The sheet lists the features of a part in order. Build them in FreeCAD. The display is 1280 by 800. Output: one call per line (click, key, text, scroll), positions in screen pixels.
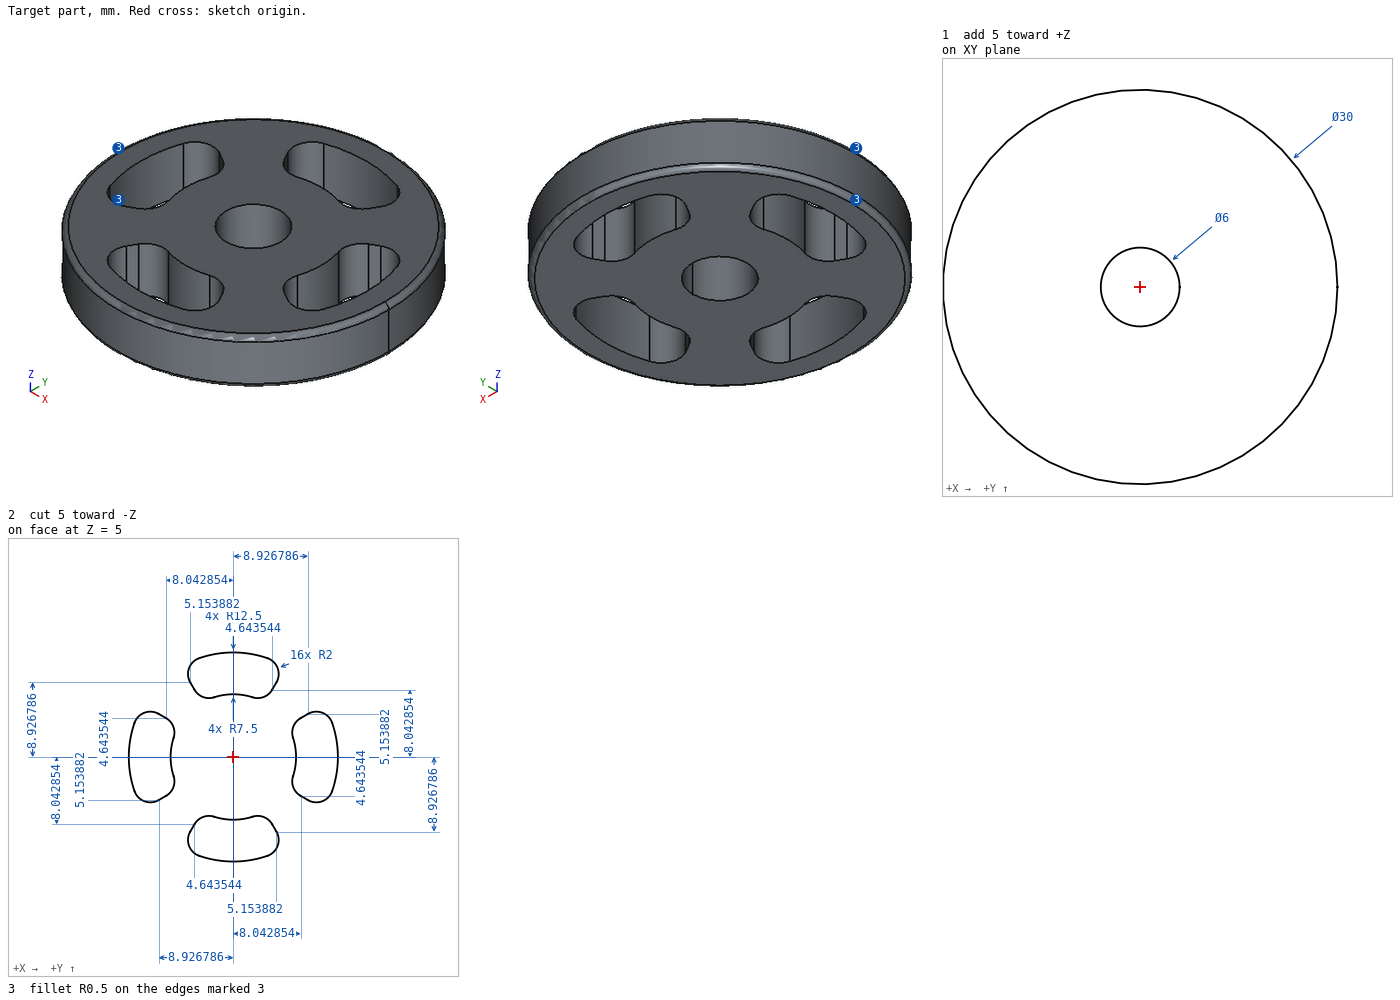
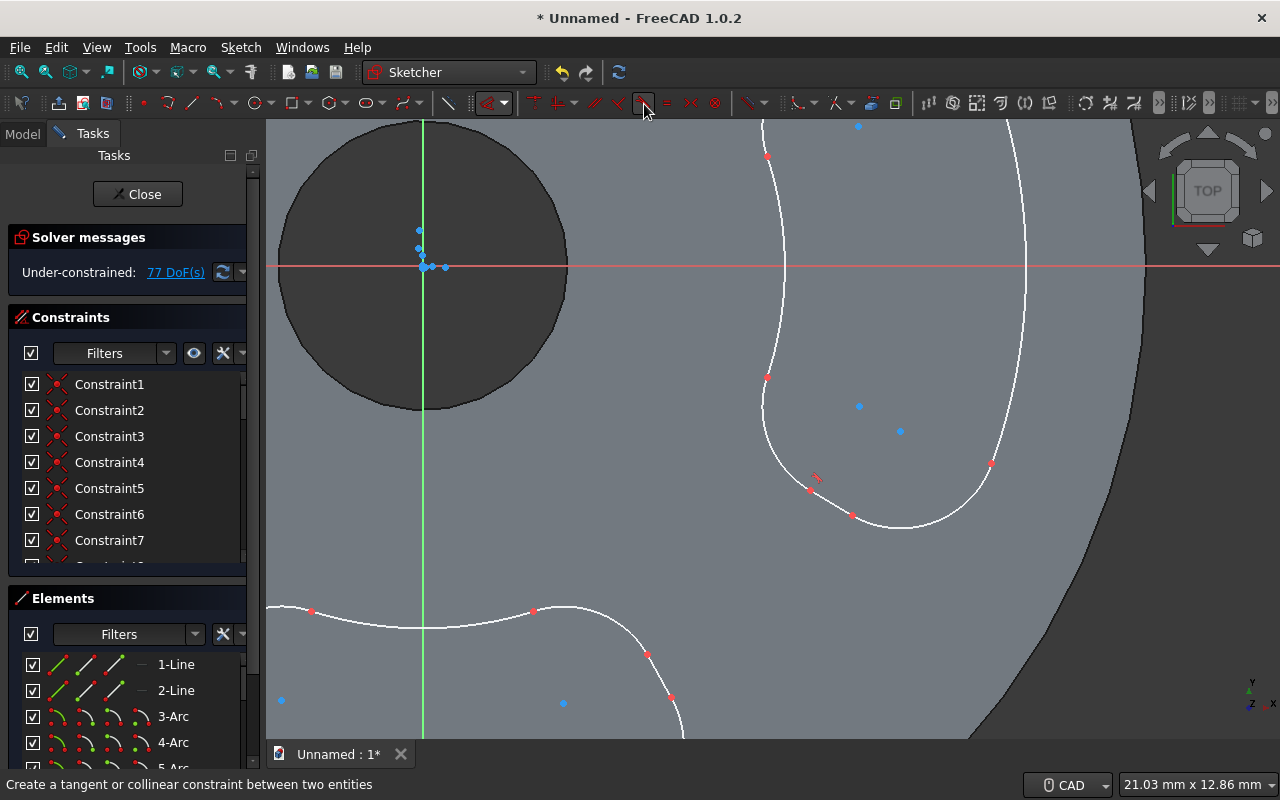
click(823, 498)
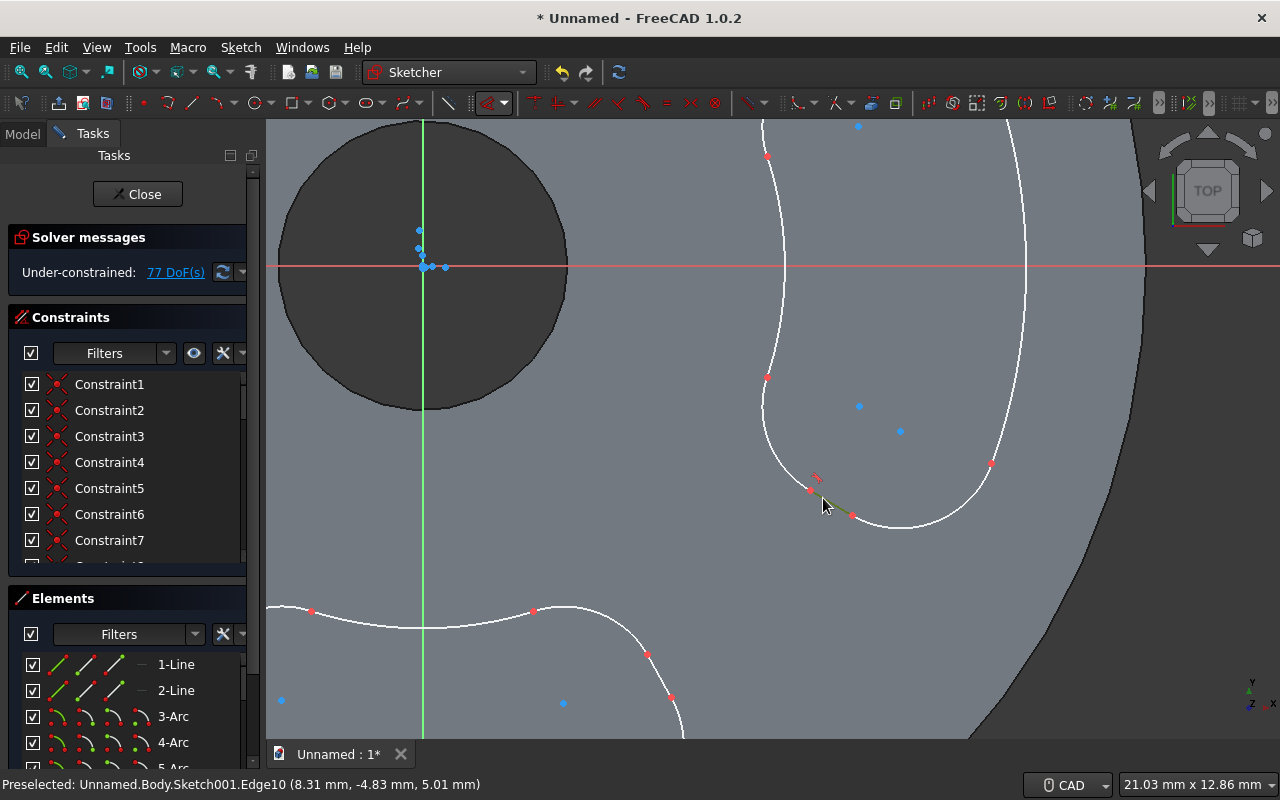
click(902, 528)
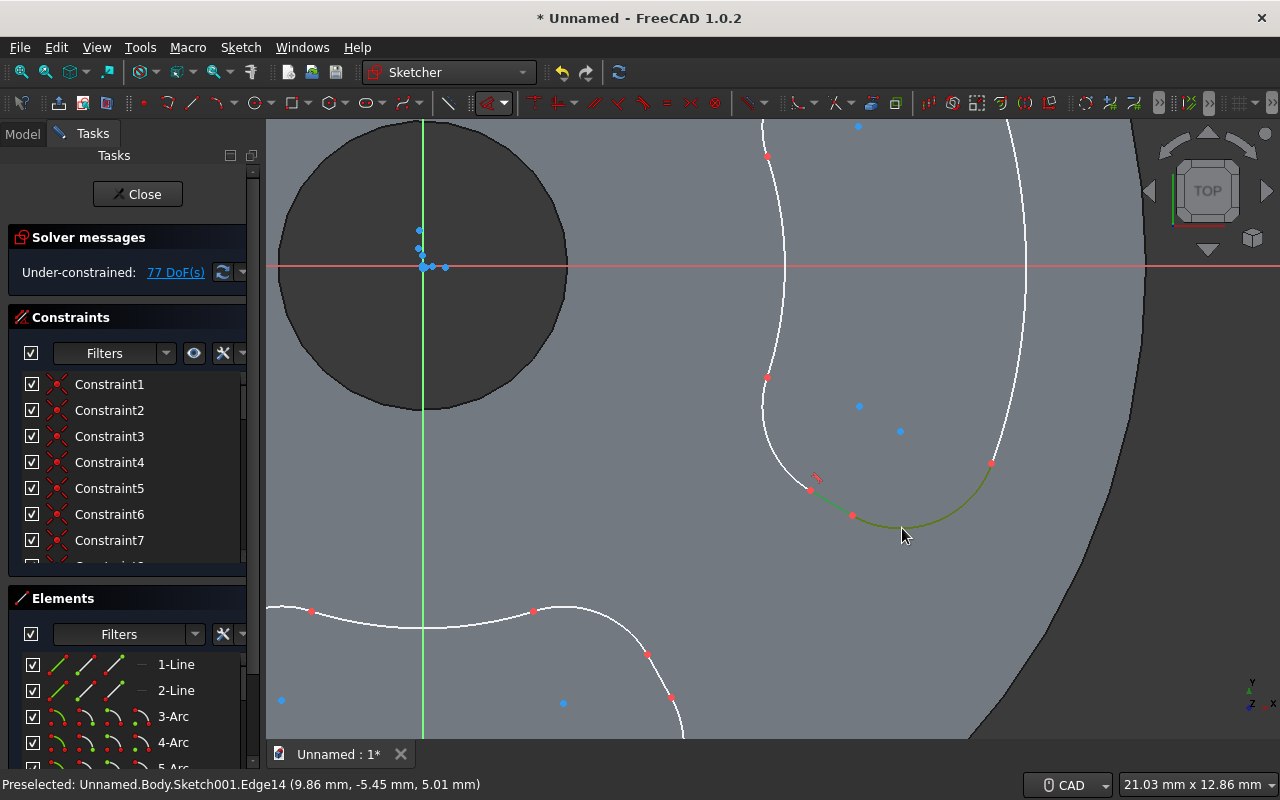
click(644, 104)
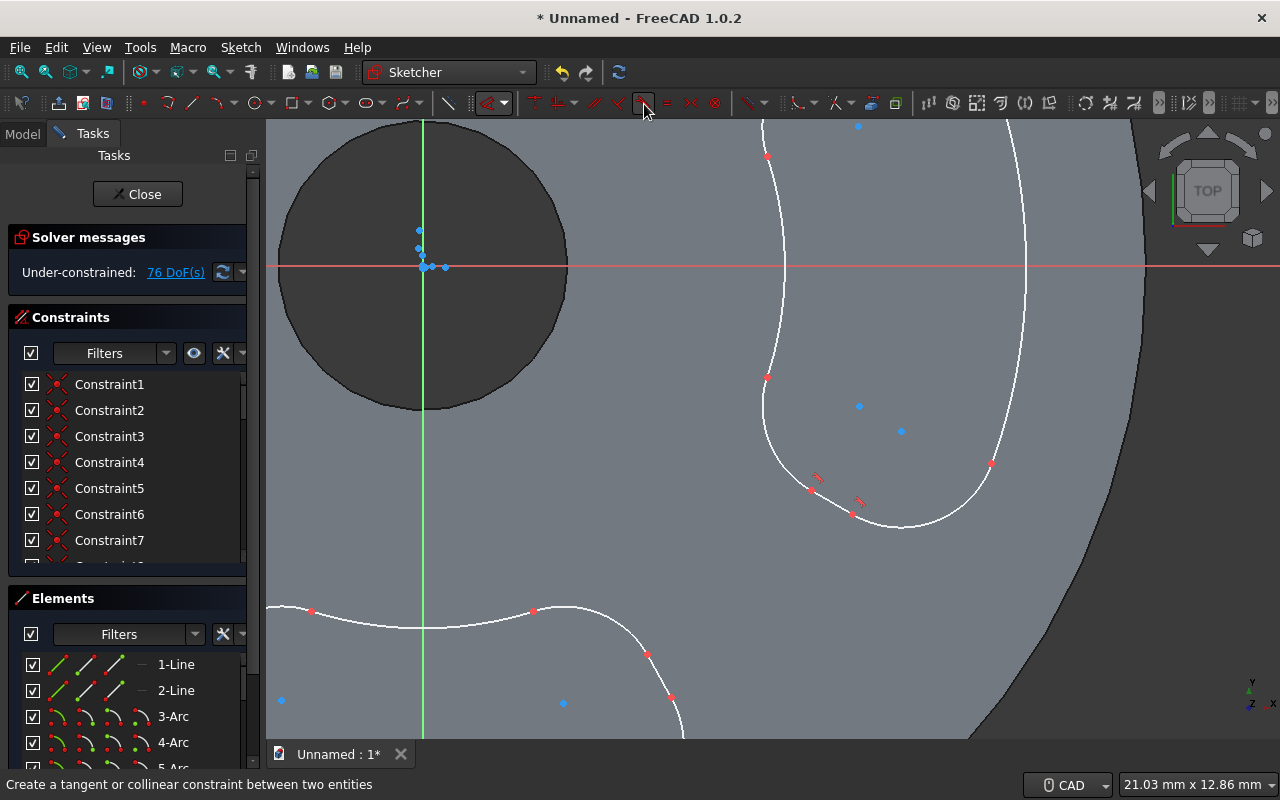
scroll(826, 499, down, 6)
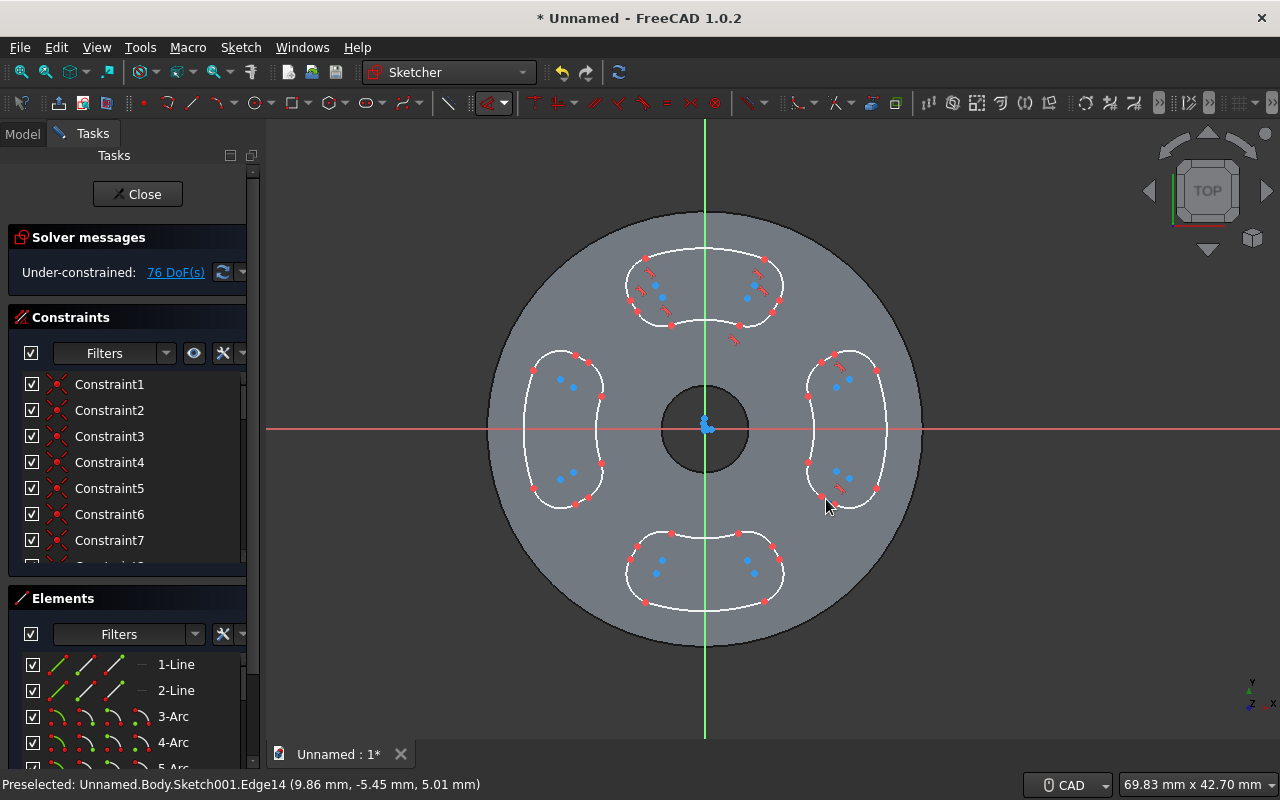
click(813, 370)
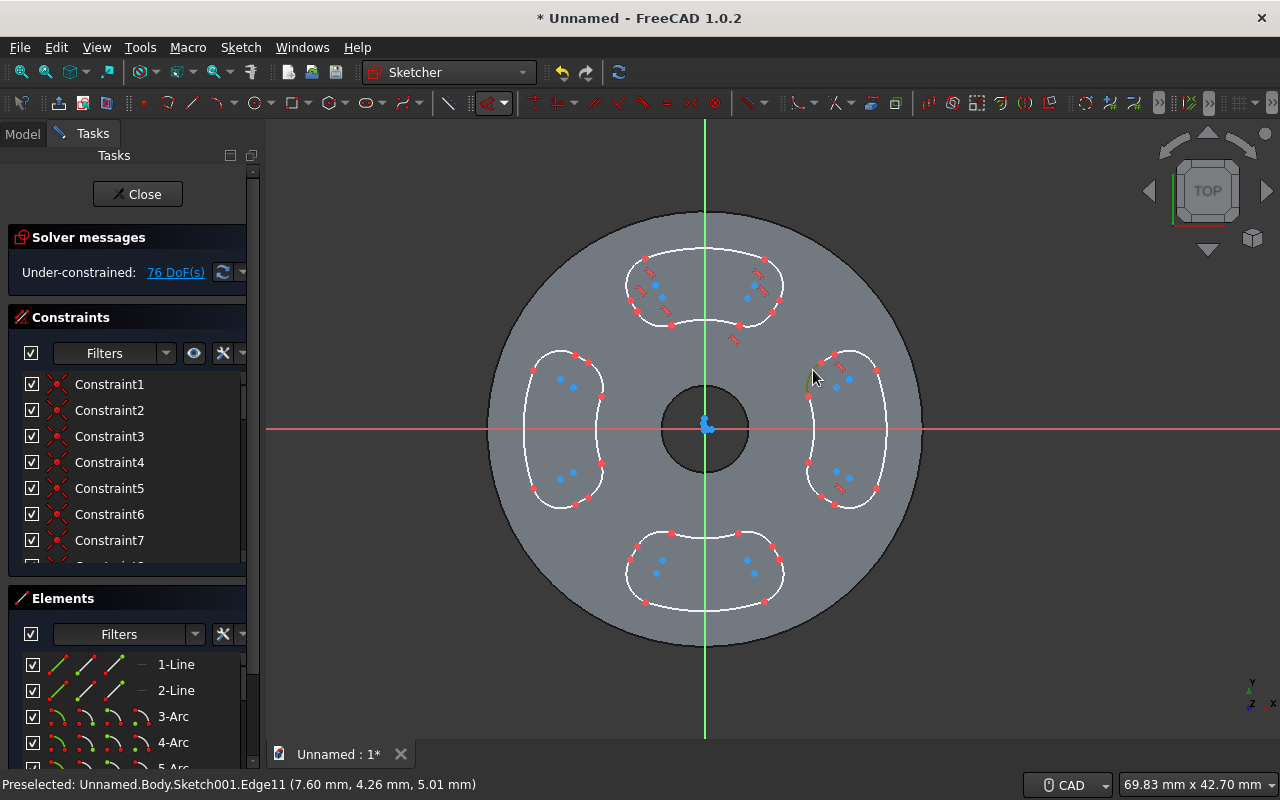
click(813, 443)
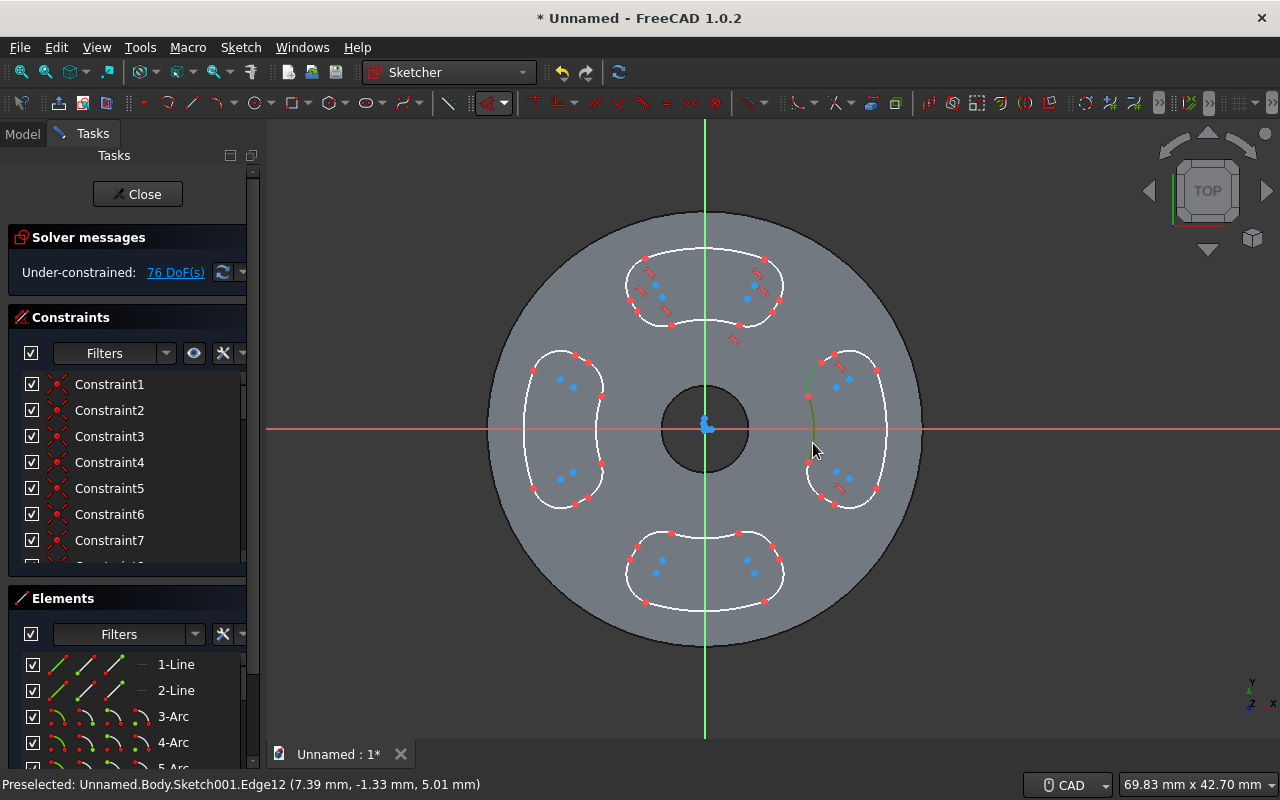
click(644, 104)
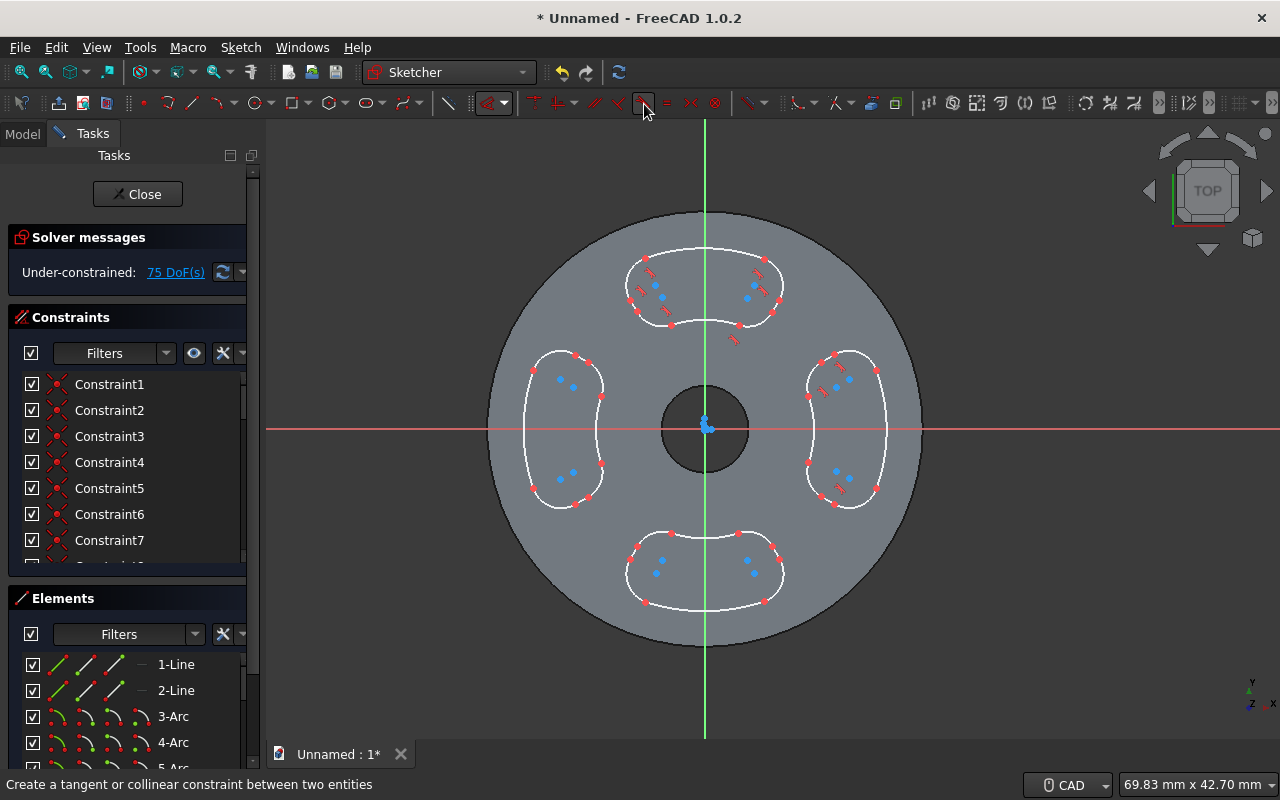
click(813, 443)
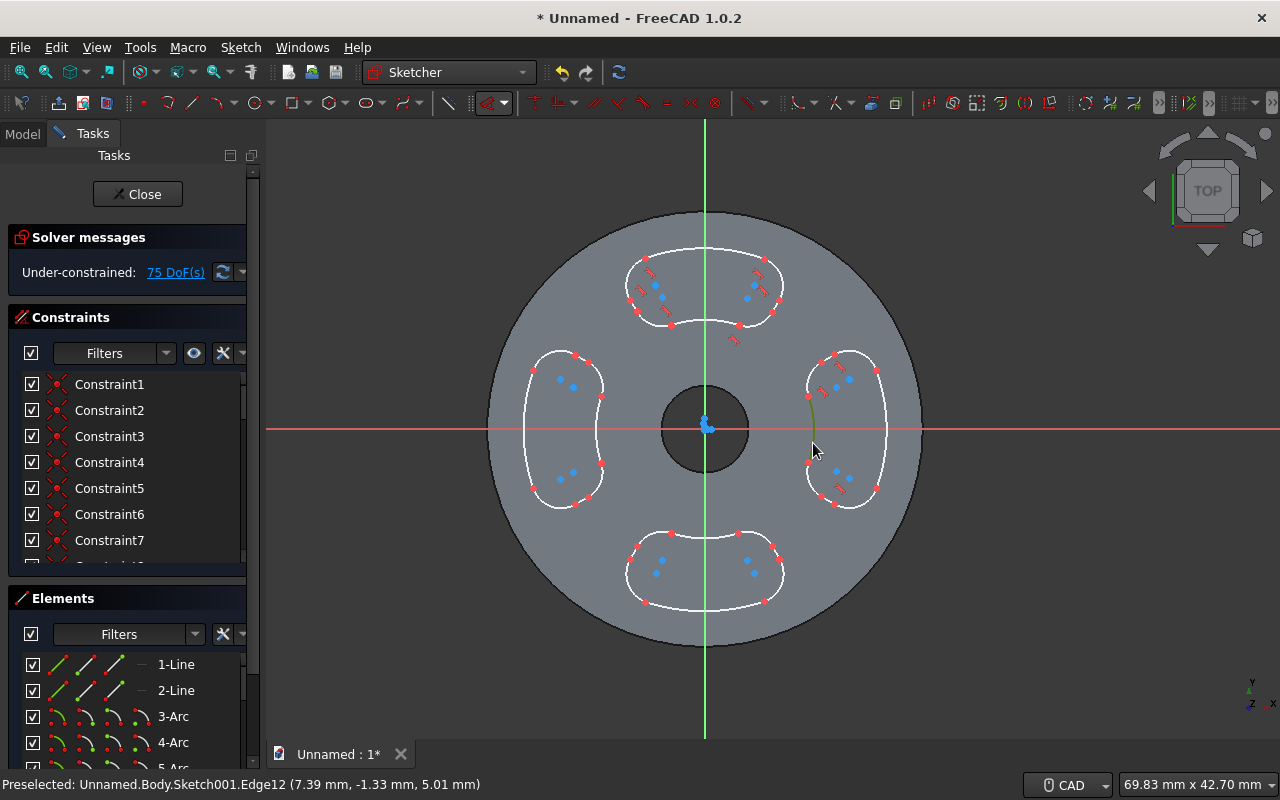
click(807, 475)